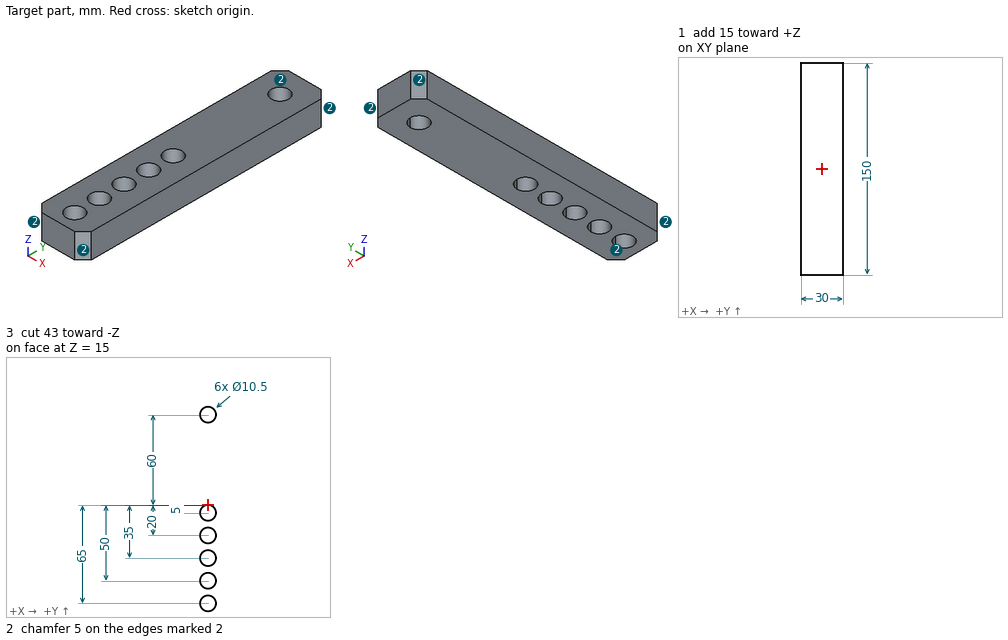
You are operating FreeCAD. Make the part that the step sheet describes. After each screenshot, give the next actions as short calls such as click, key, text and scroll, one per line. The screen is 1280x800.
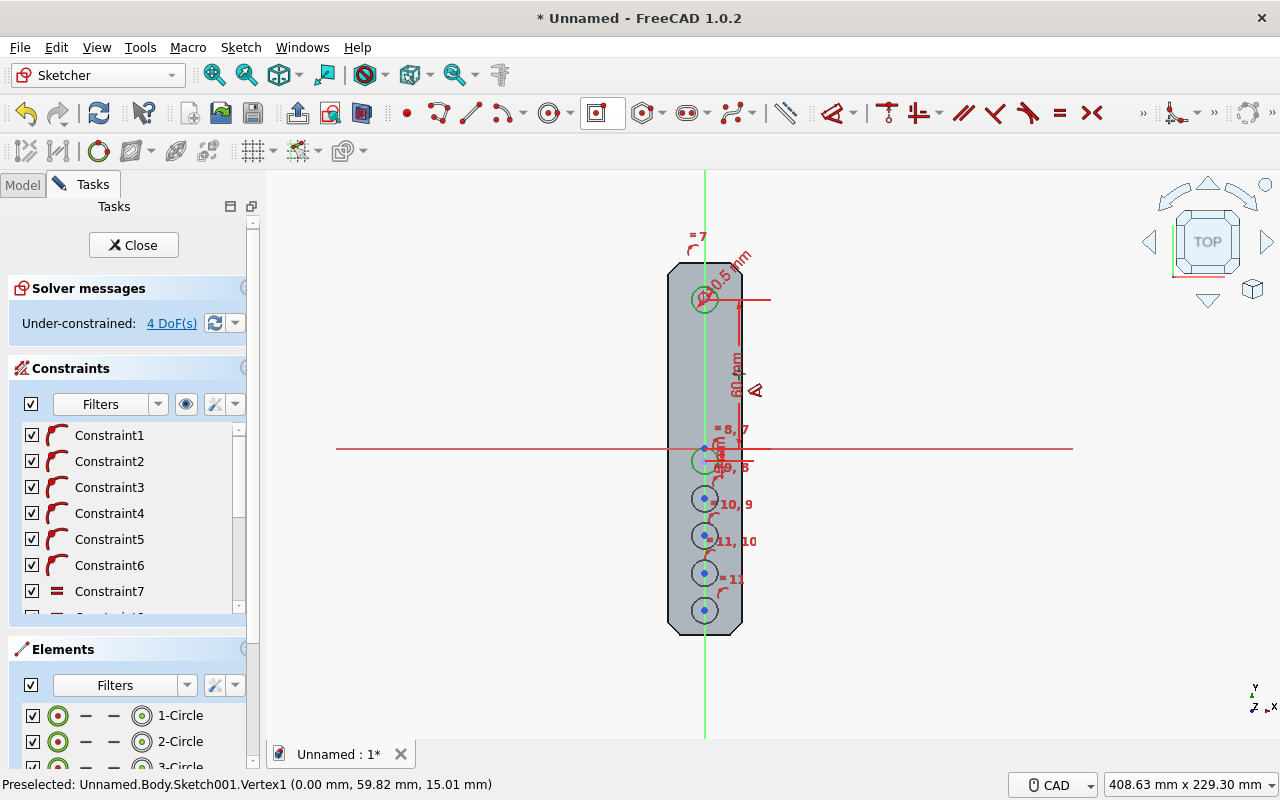
click(705, 499)
click(739, 485)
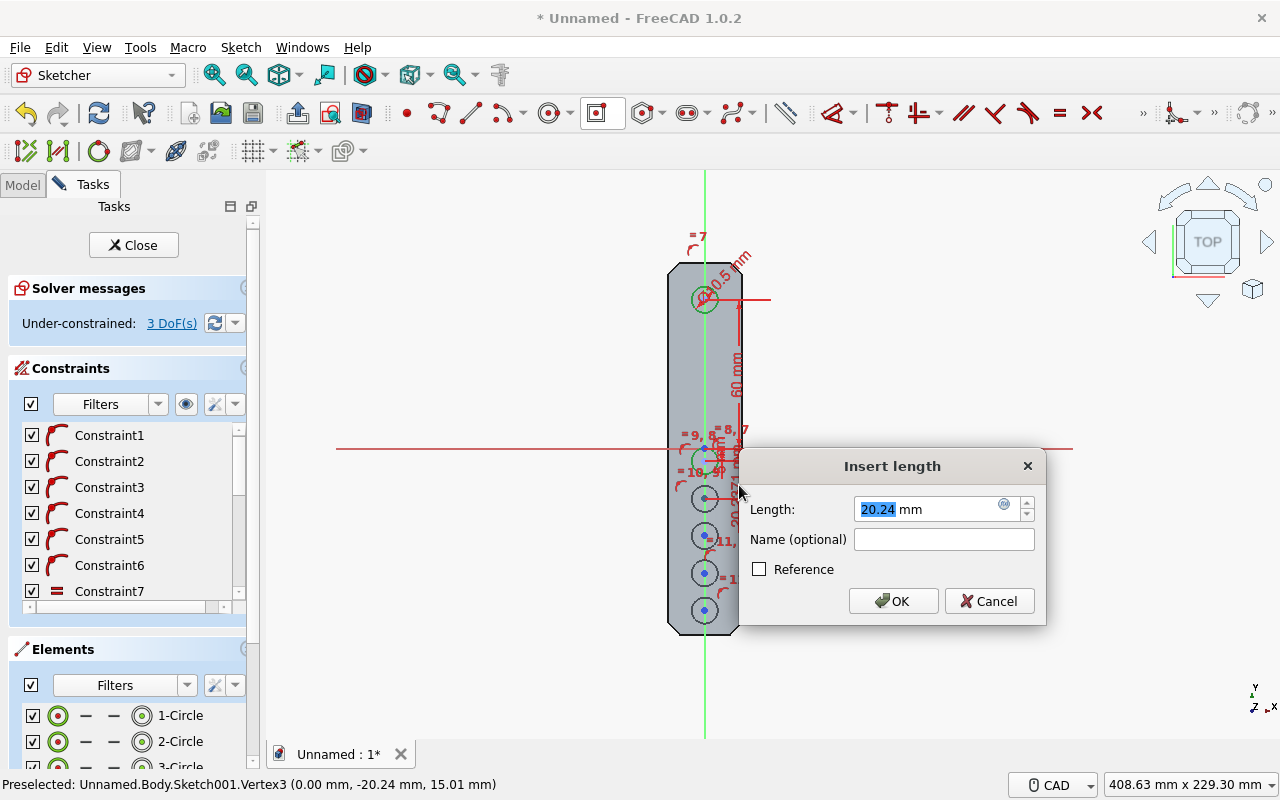
text(20)
key(Return)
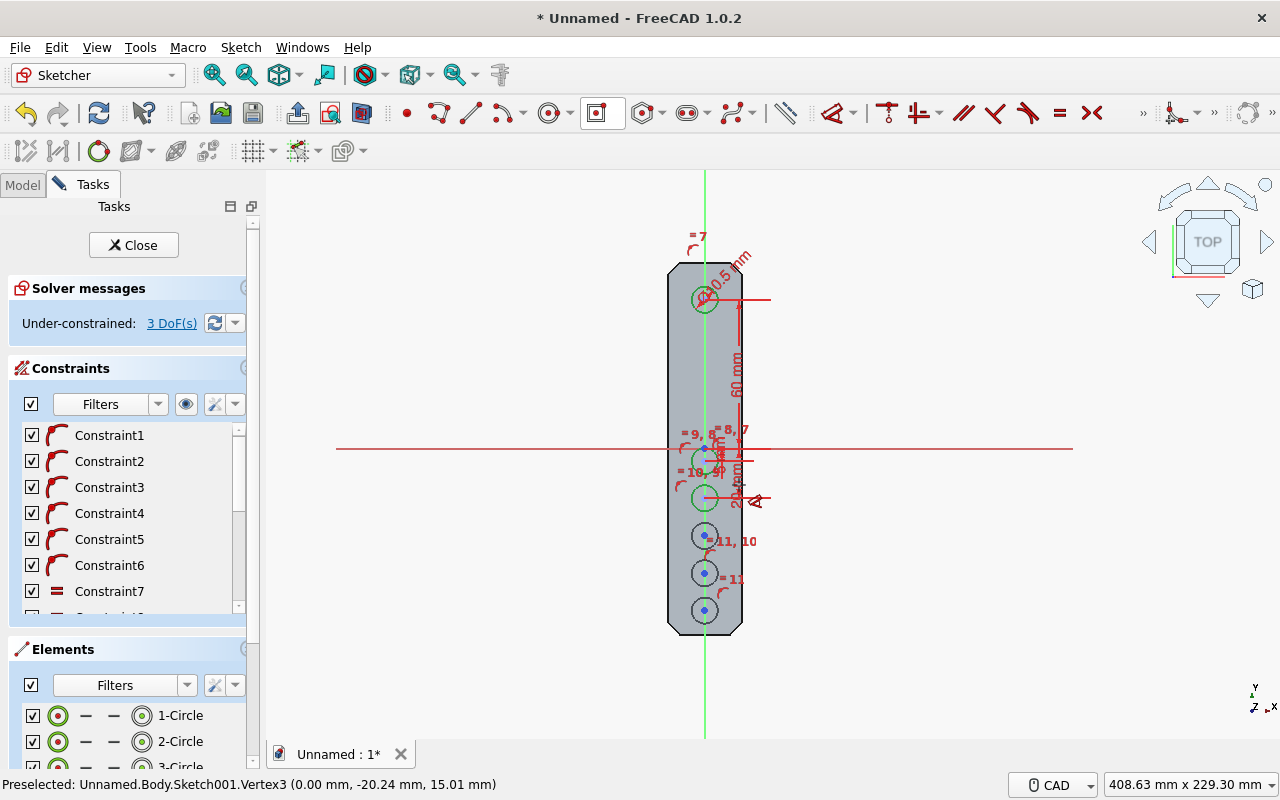
click(705, 536)
click(739, 512)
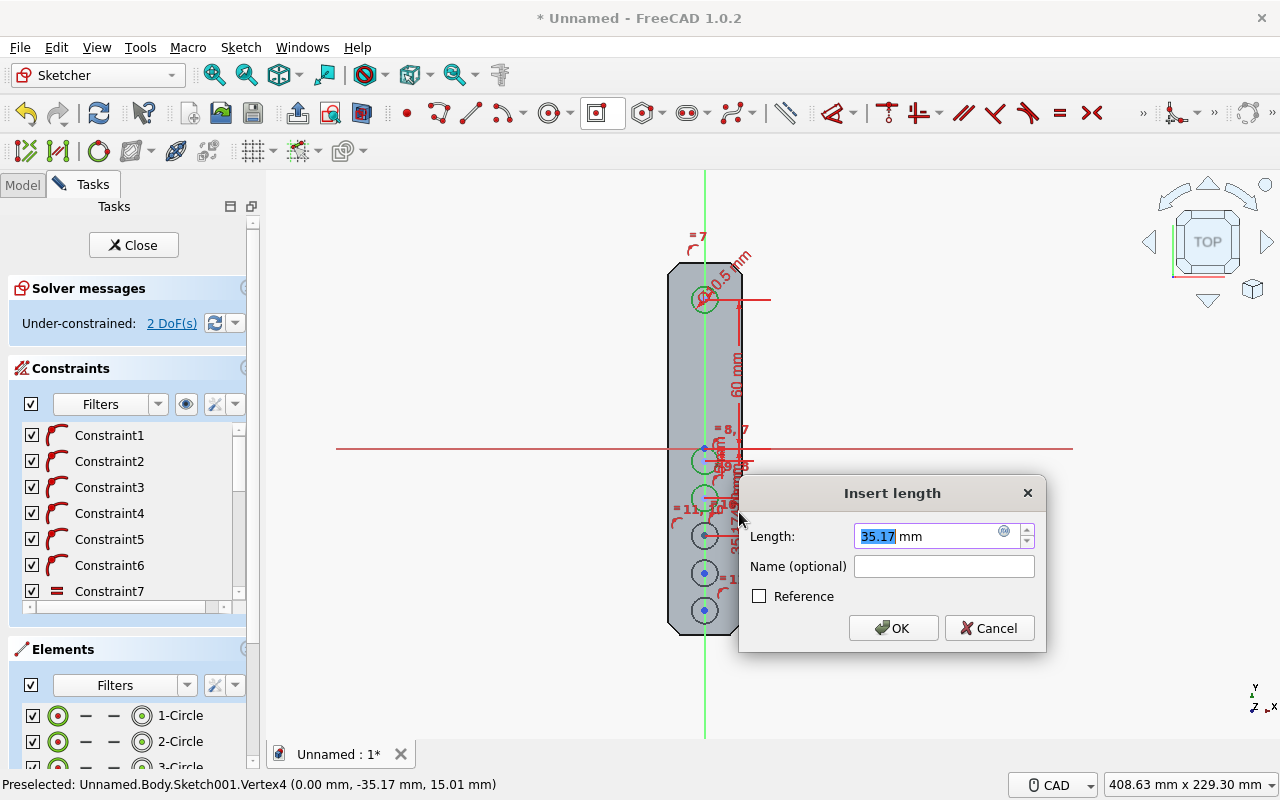
text(35)
key(Return)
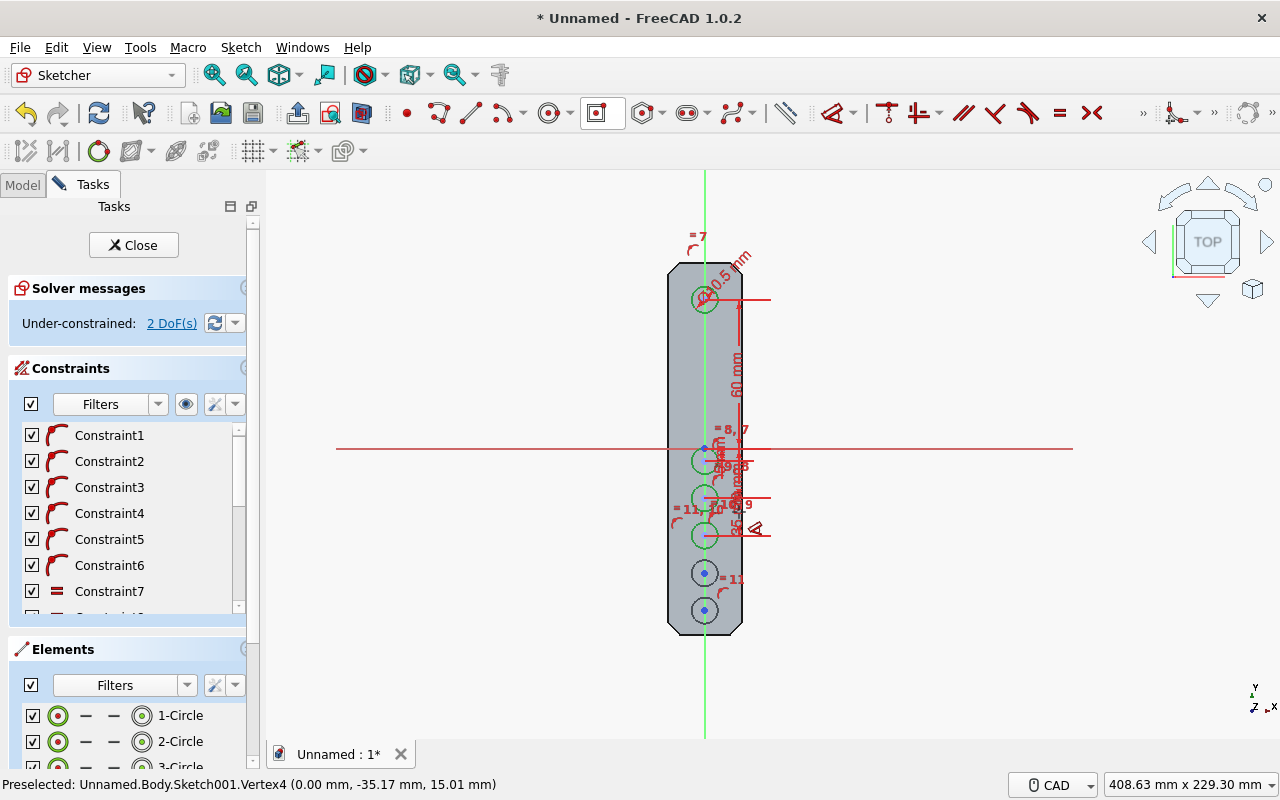
click(705, 573)
click(739, 540)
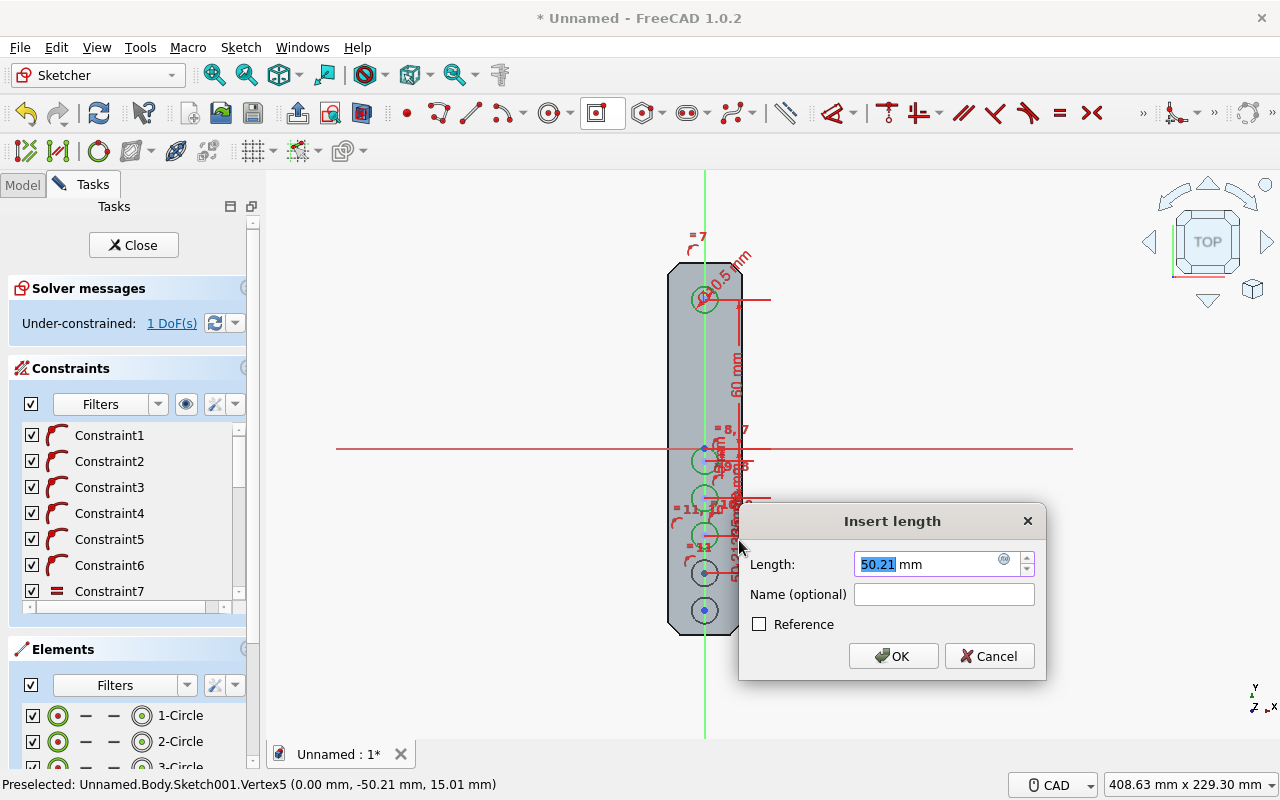
text(50)
key(Return)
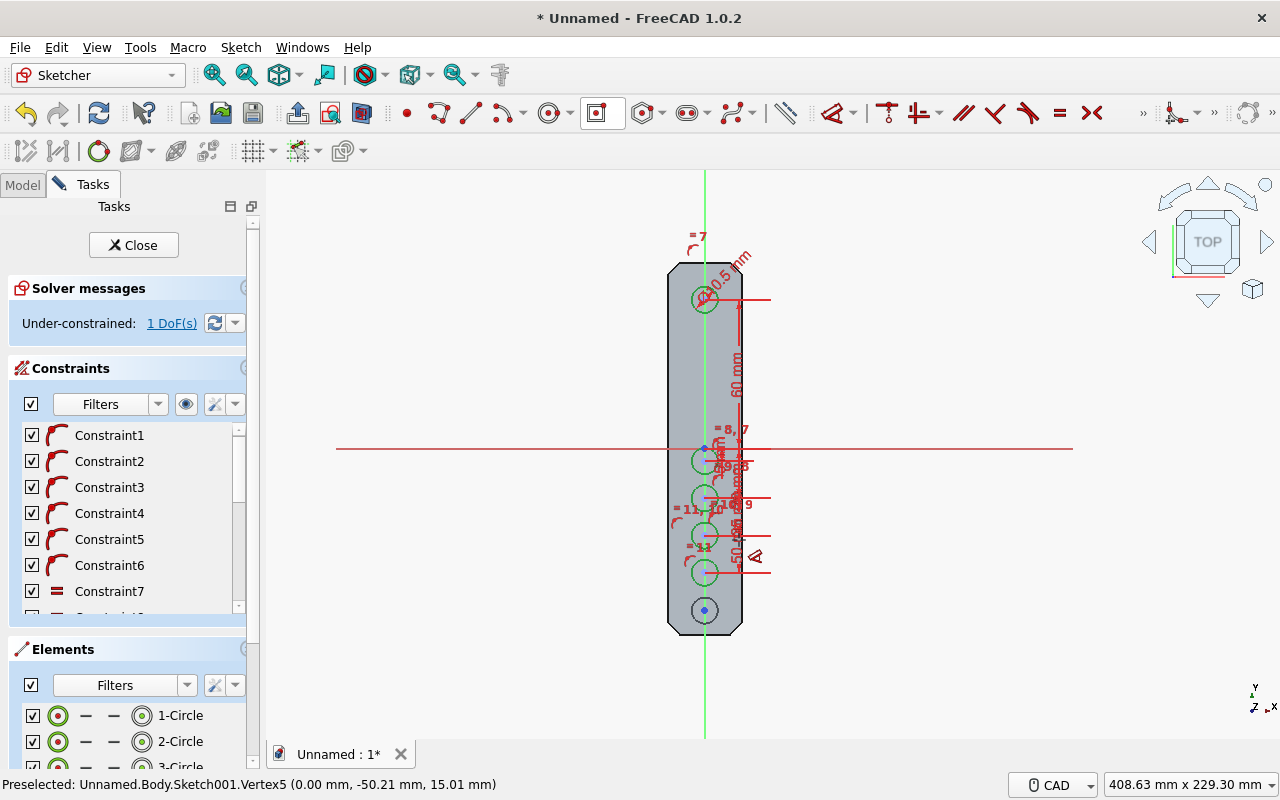
click(705, 611)
click(739, 567)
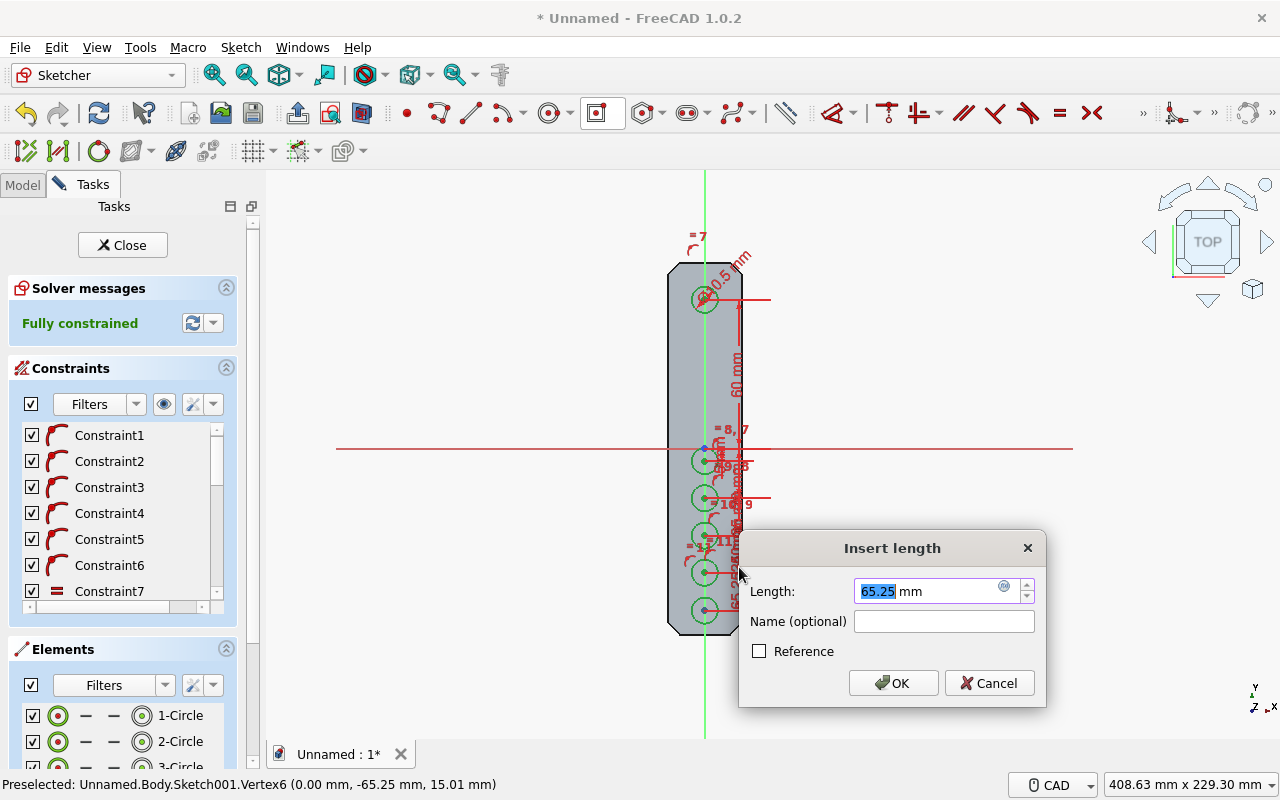
text(65)
key(Return)
key(Escape)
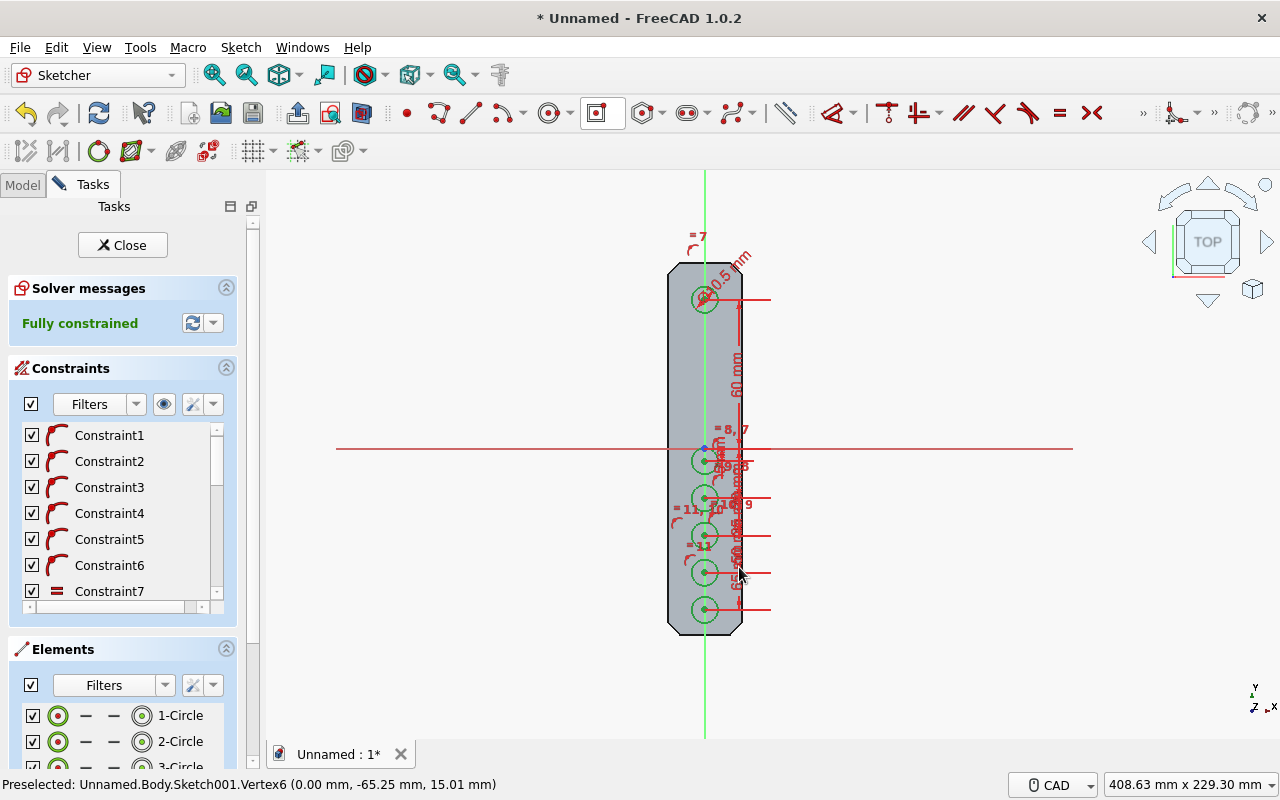
click(123, 245)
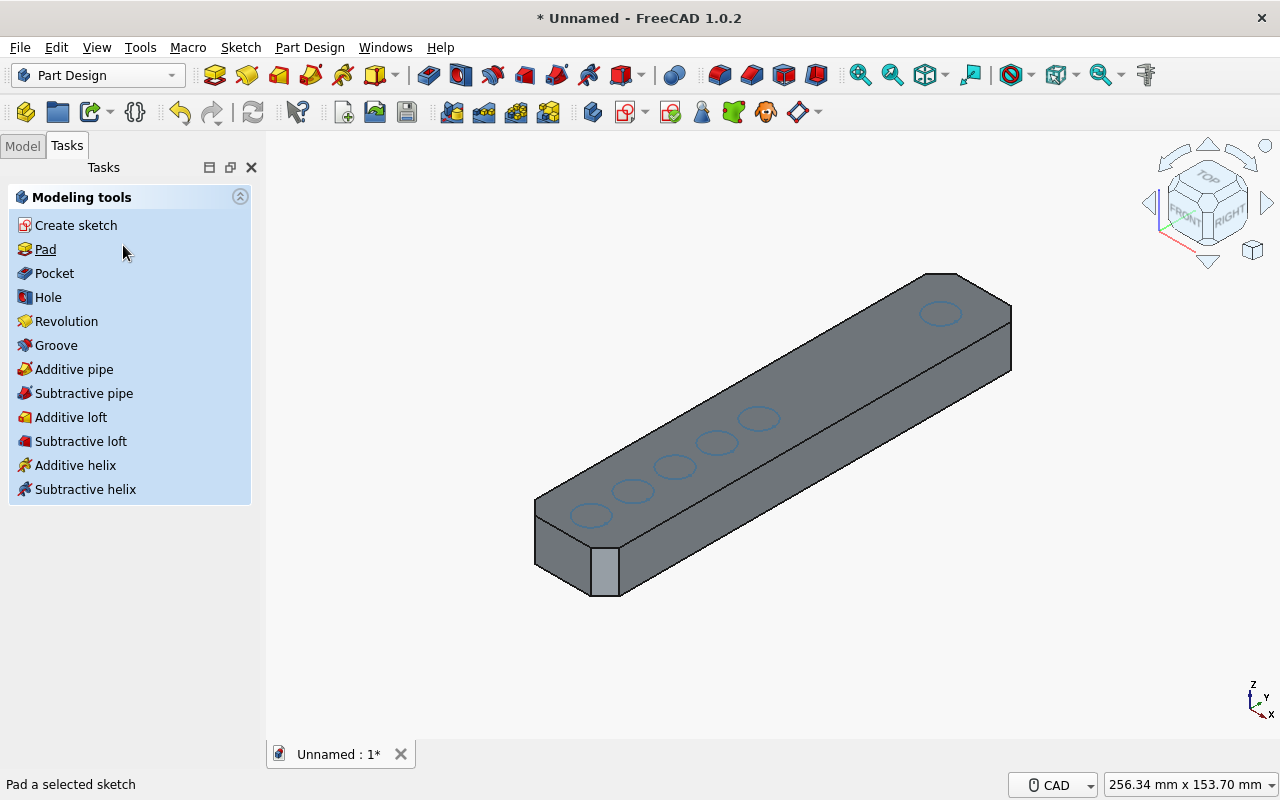
click(430, 76)